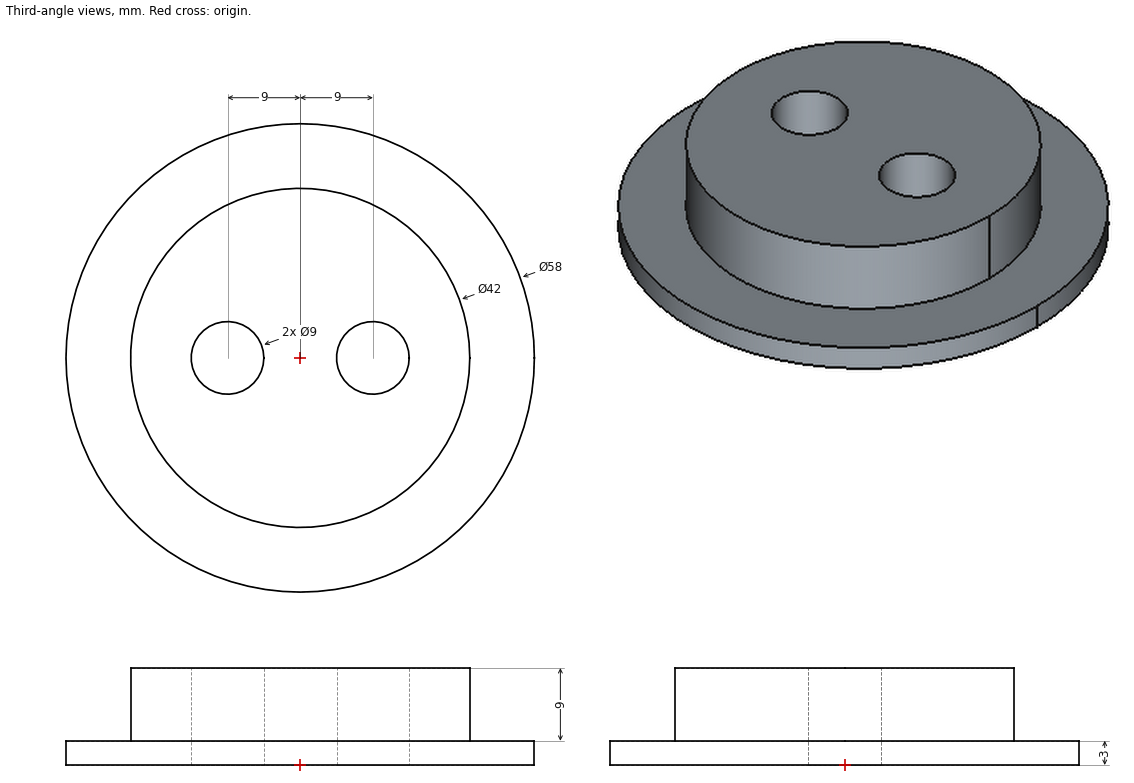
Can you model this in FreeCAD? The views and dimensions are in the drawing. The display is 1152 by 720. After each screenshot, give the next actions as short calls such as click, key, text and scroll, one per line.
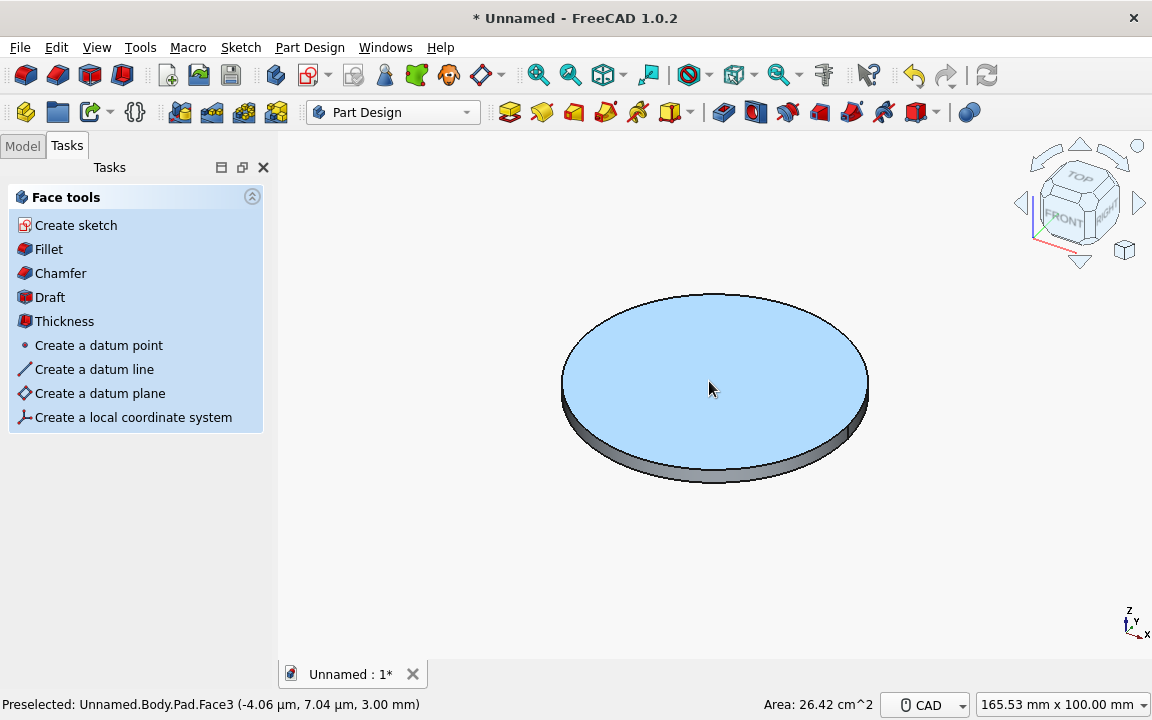
click(308, 76)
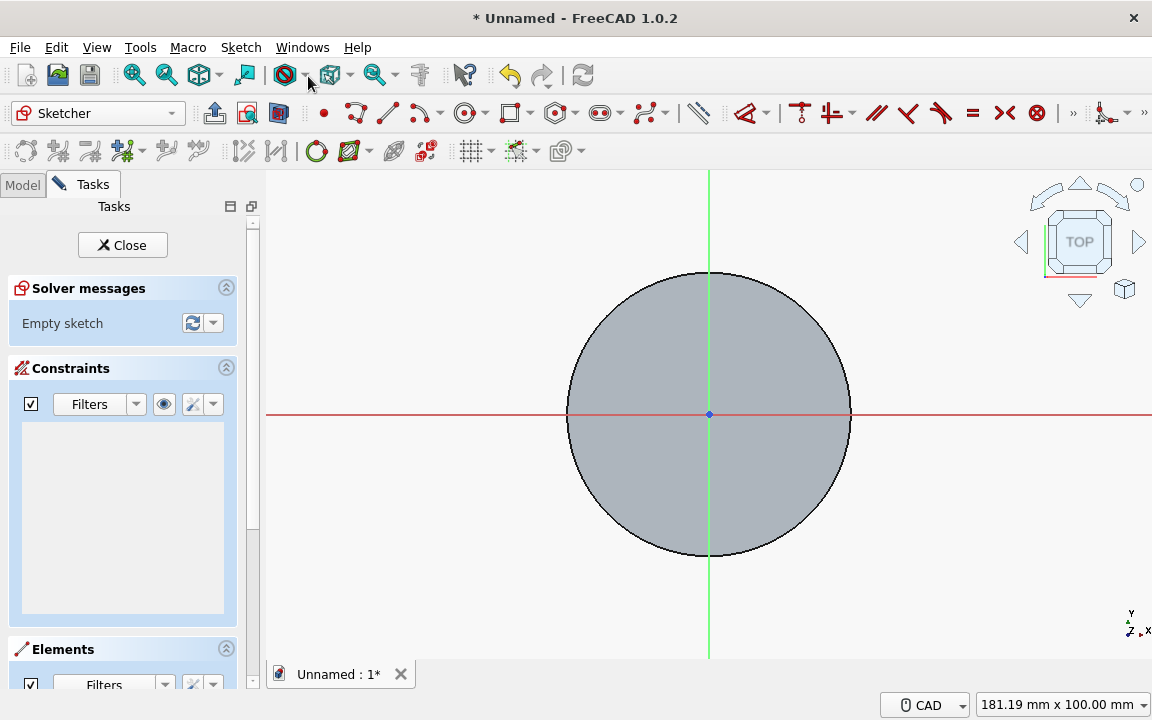
scroll(848, 414, up, 2)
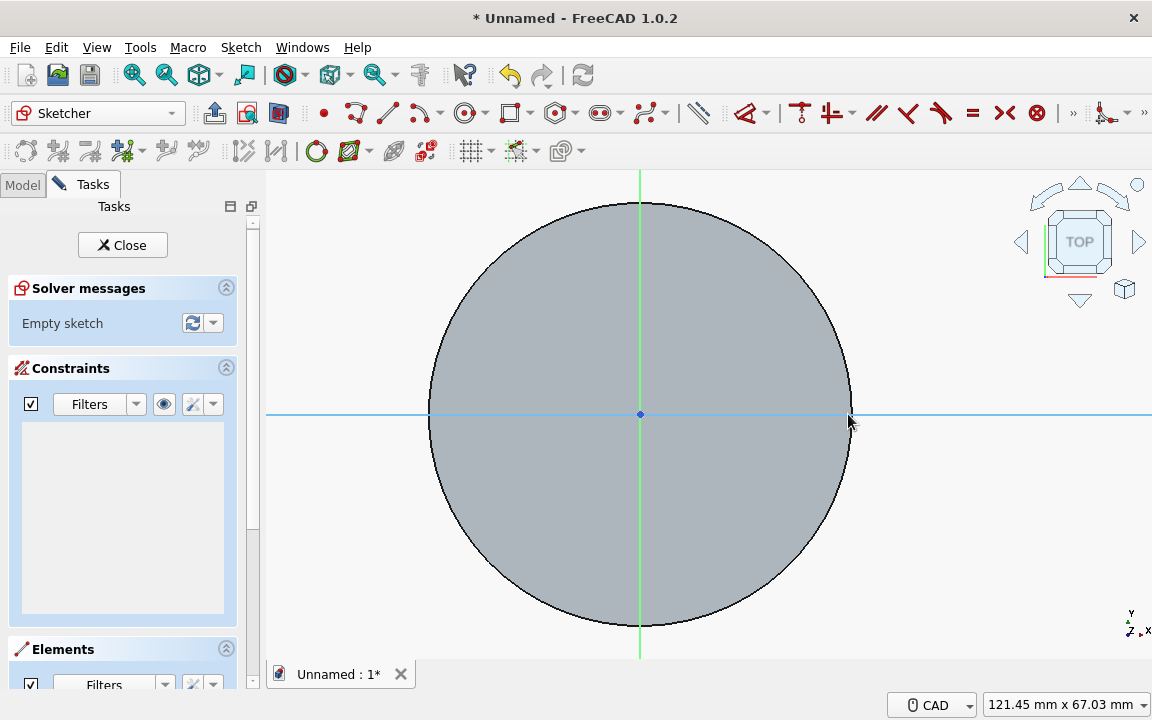
click(466, 114)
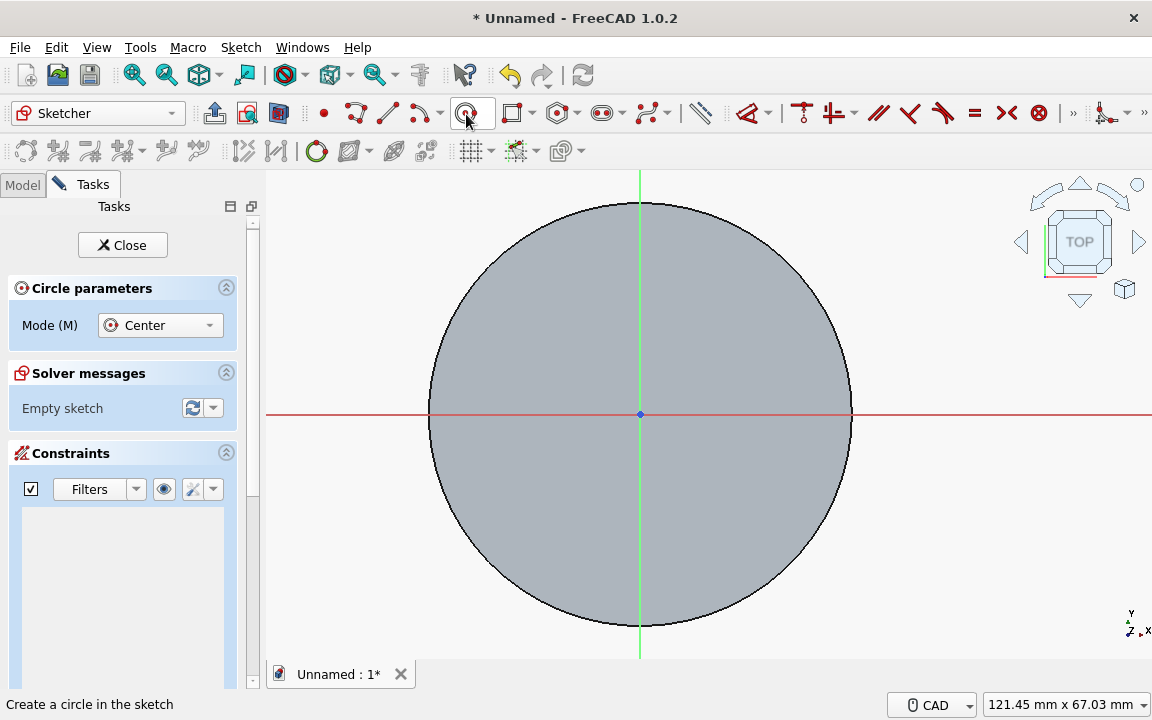
click(640, 414)
move(749, 306)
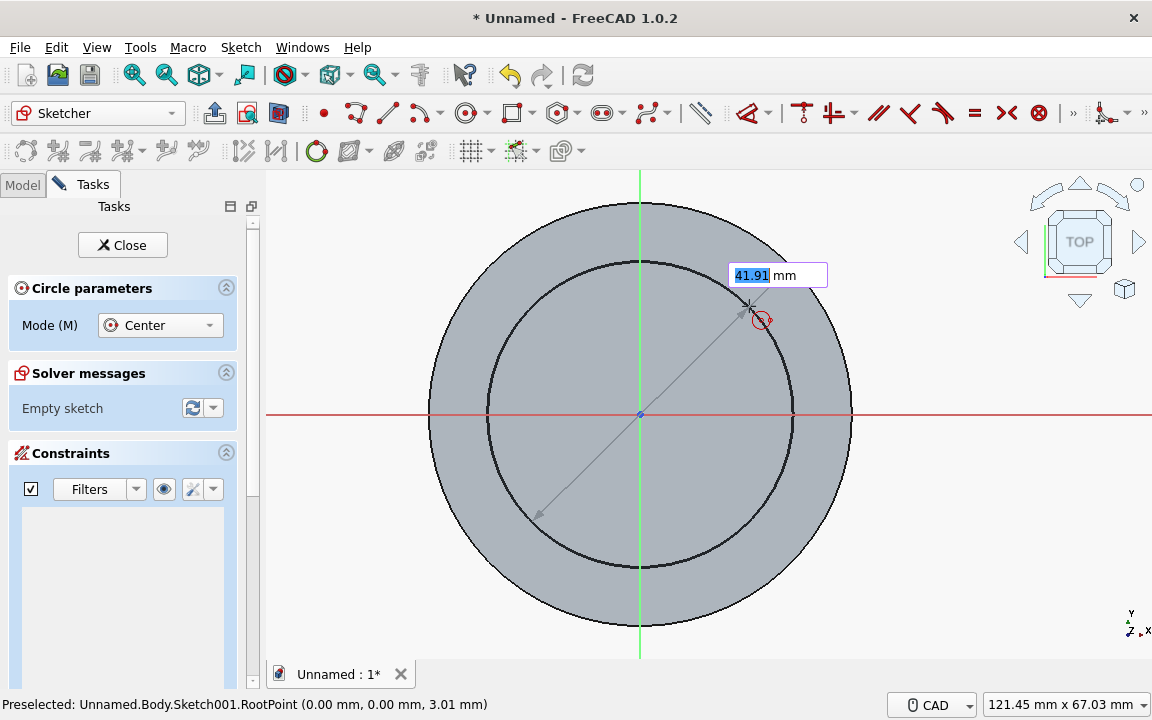
text(42)
key(Return)
key(Escape)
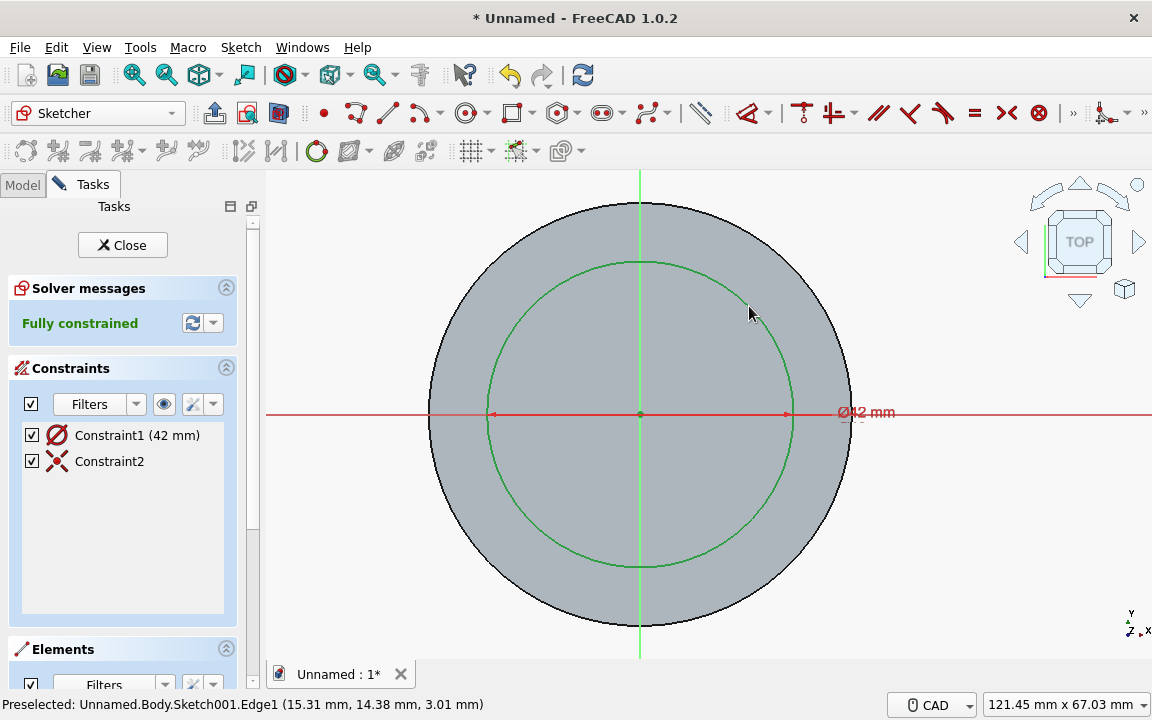
click(123, 245)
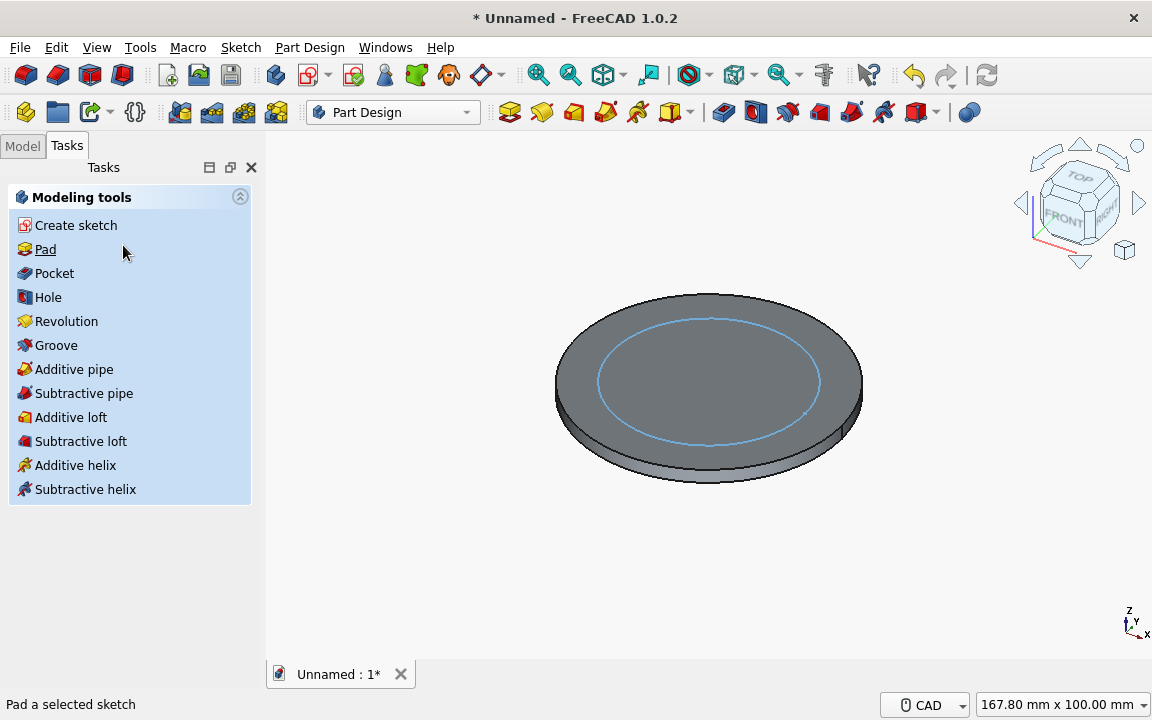
click(510, 112)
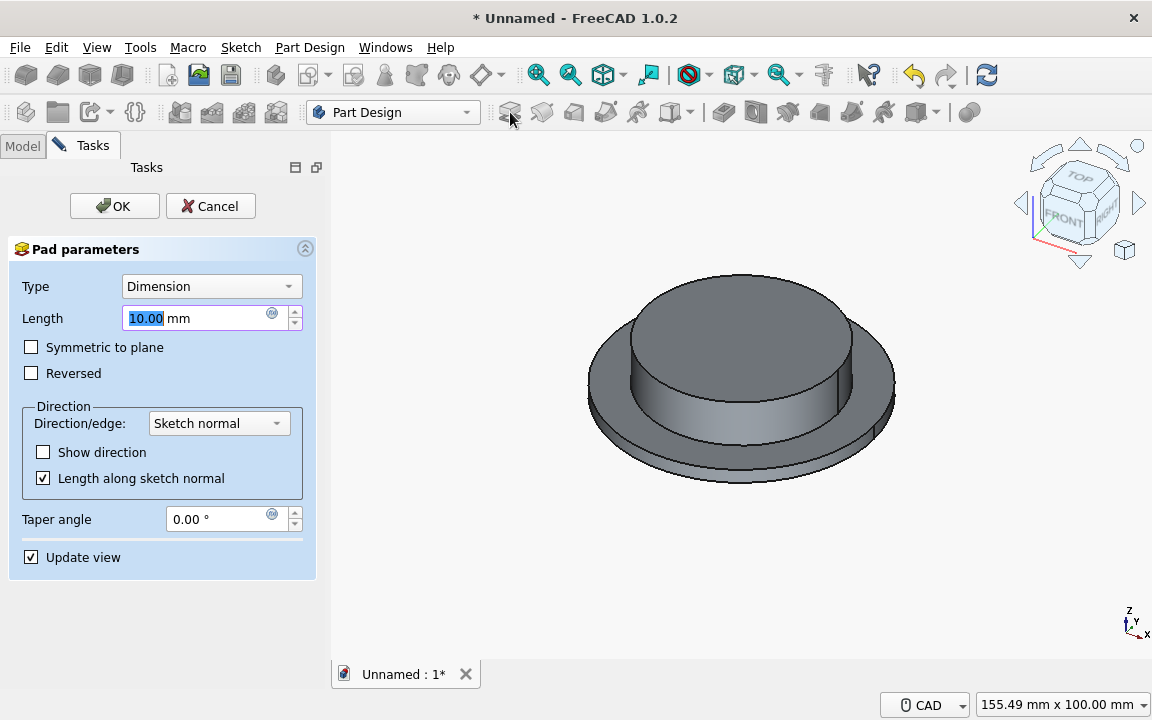
text(9)
key(Tab)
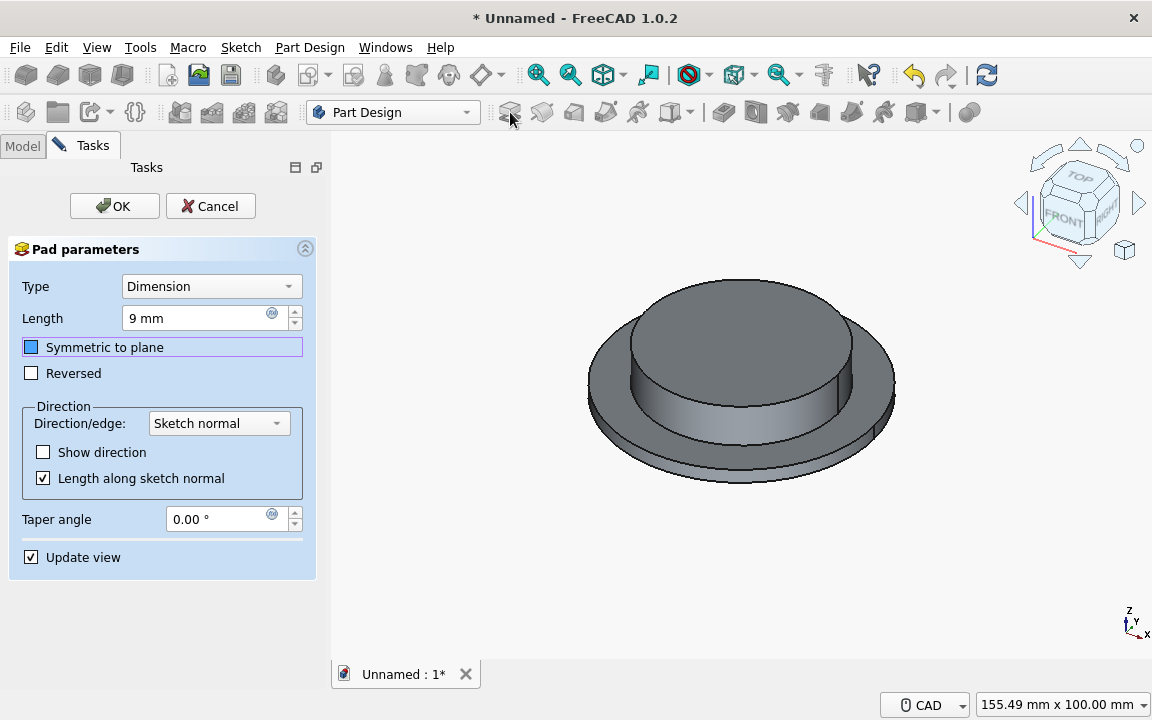
click(115, 206)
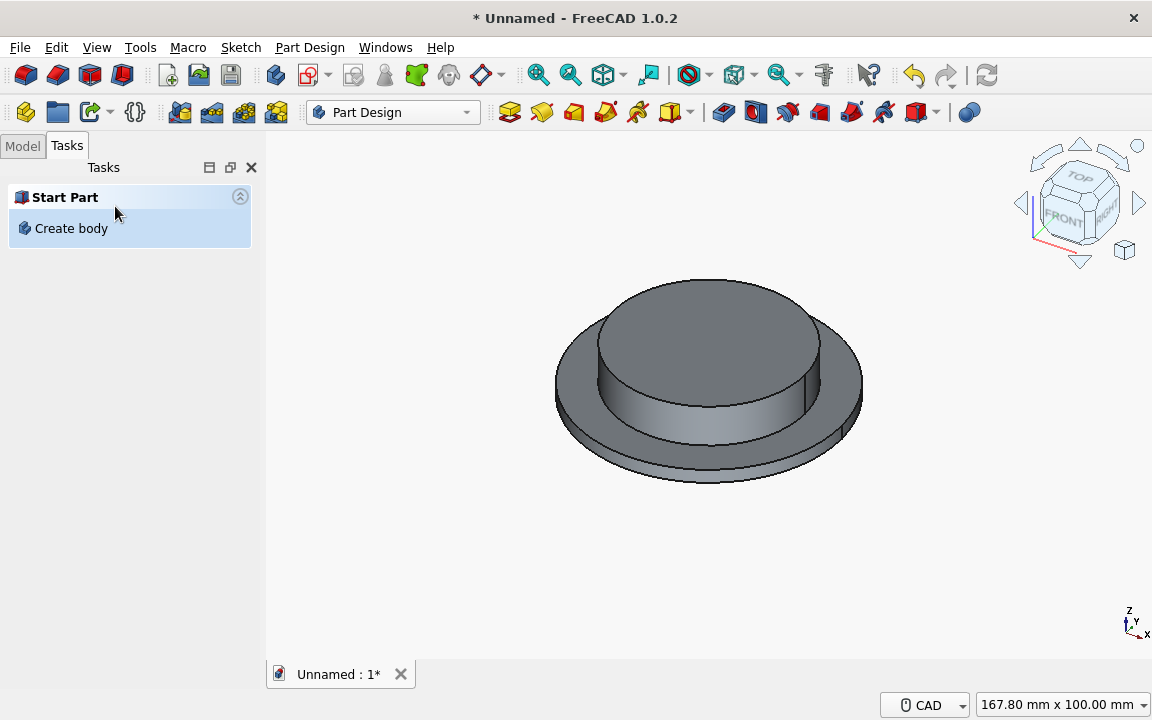
click(709, 342)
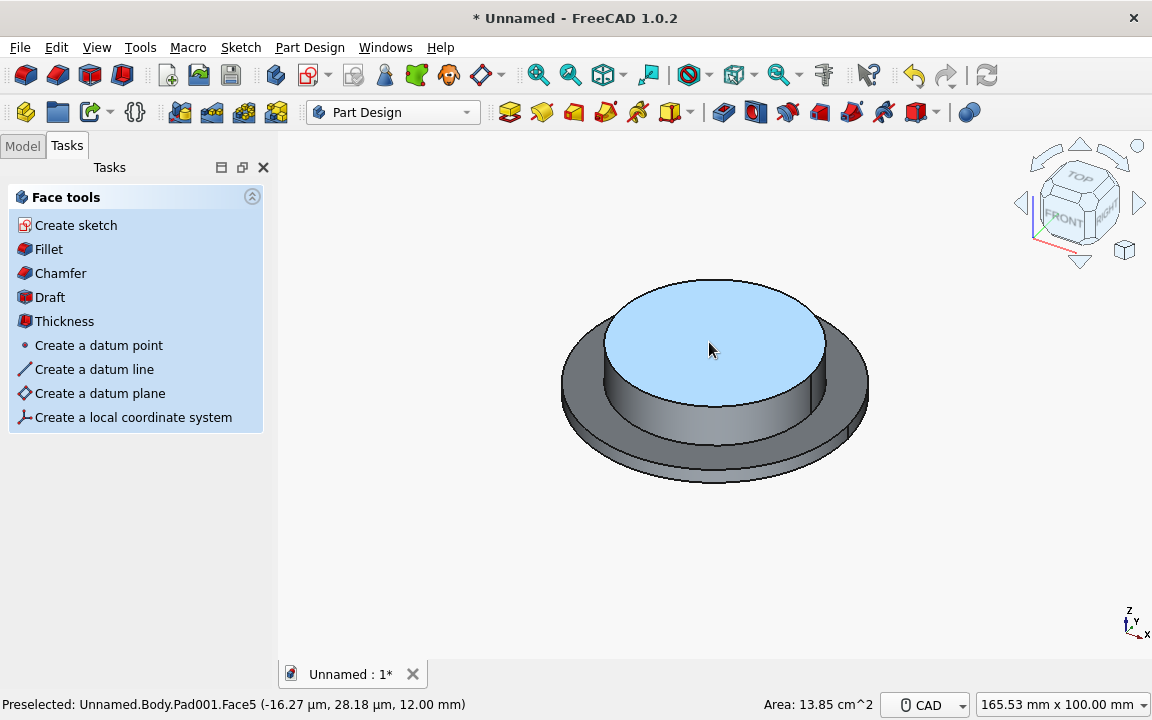
click(308, 76)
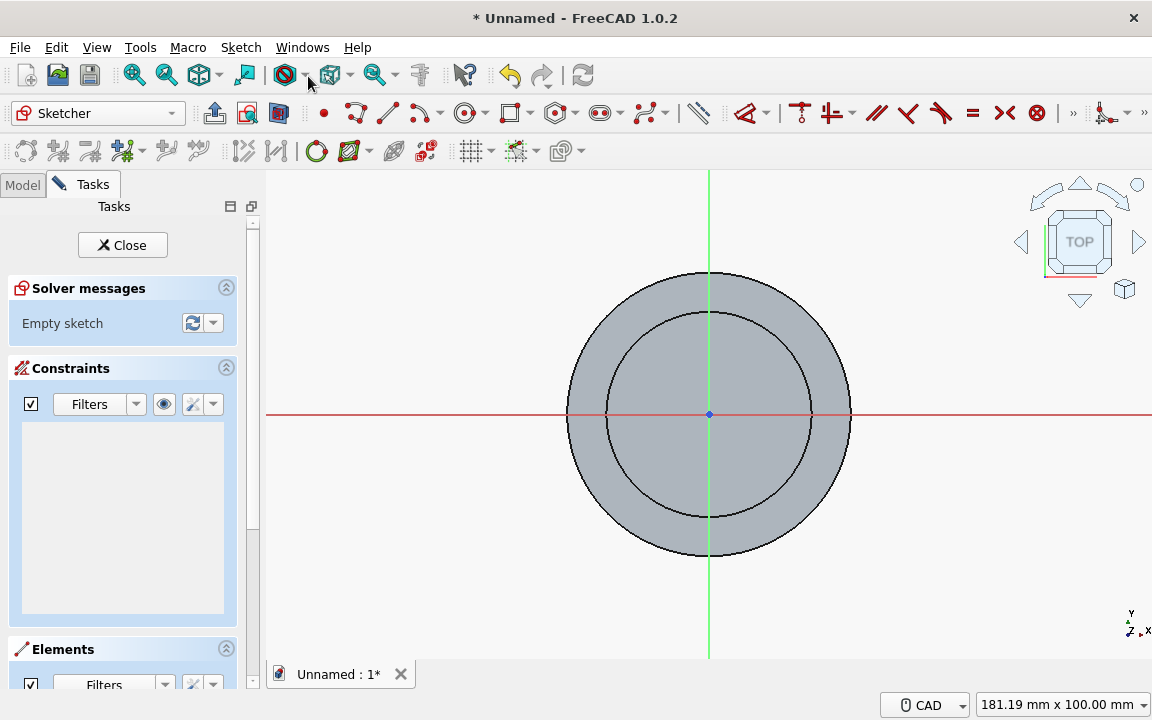
scroll(731, 415, up, 7)